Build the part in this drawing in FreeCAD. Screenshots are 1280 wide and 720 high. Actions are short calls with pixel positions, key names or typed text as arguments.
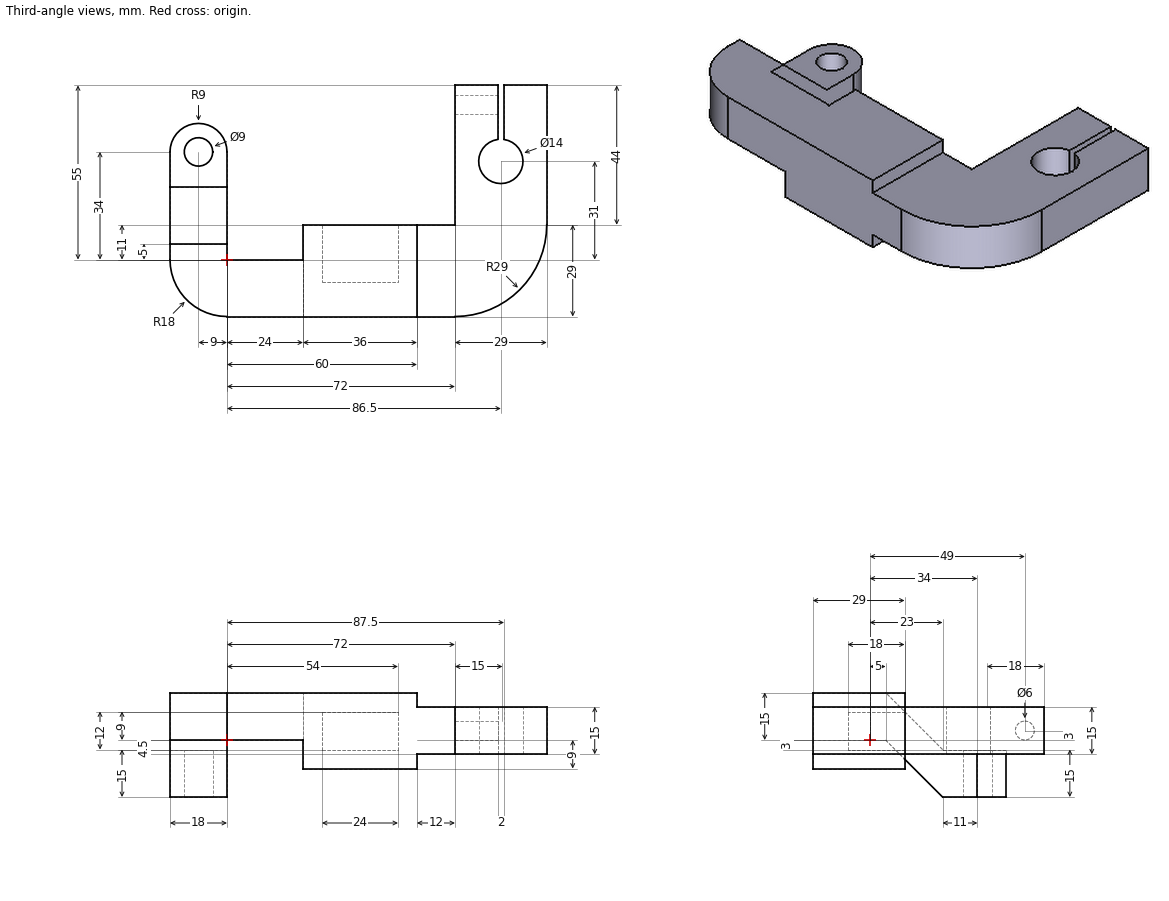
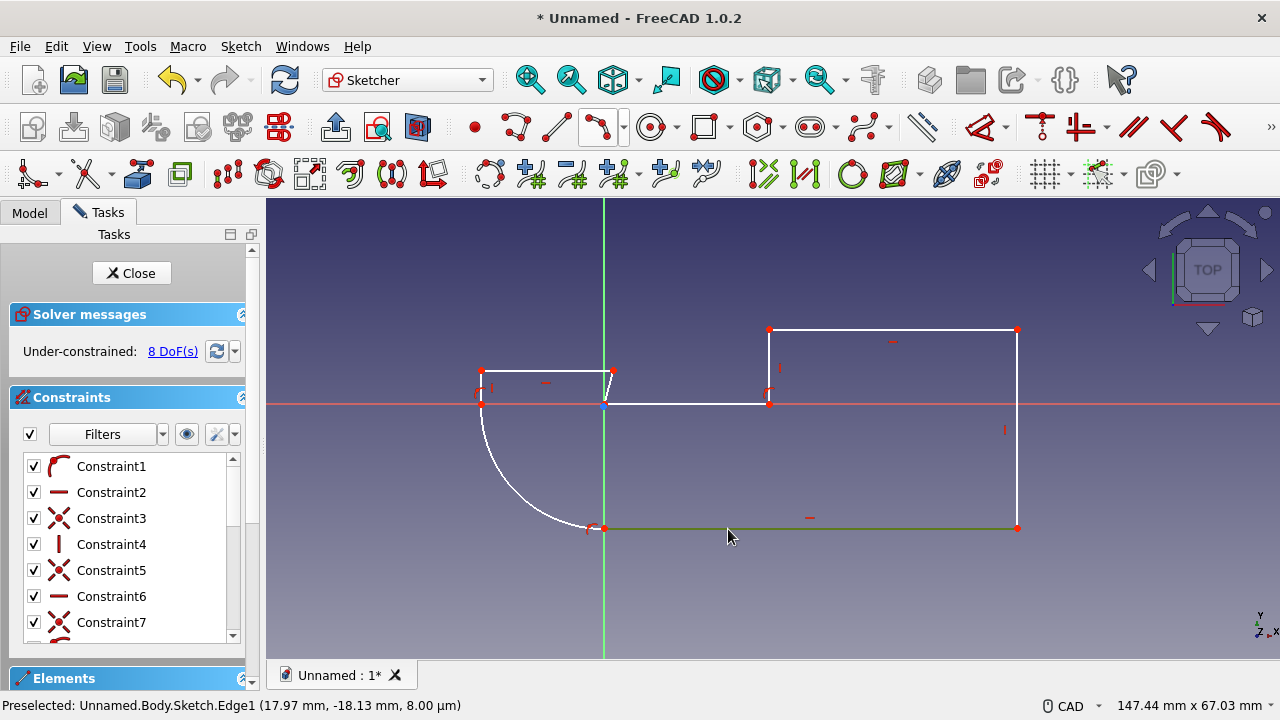
click(494, 461)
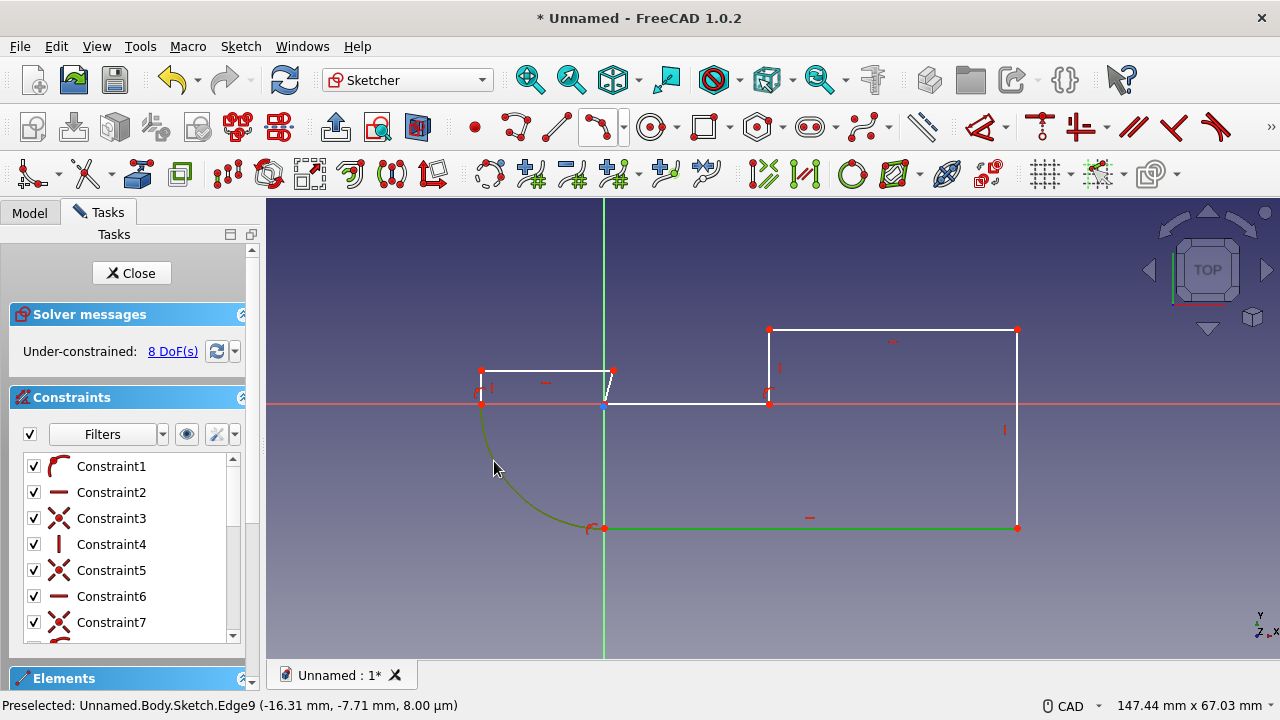
click(1216, 128)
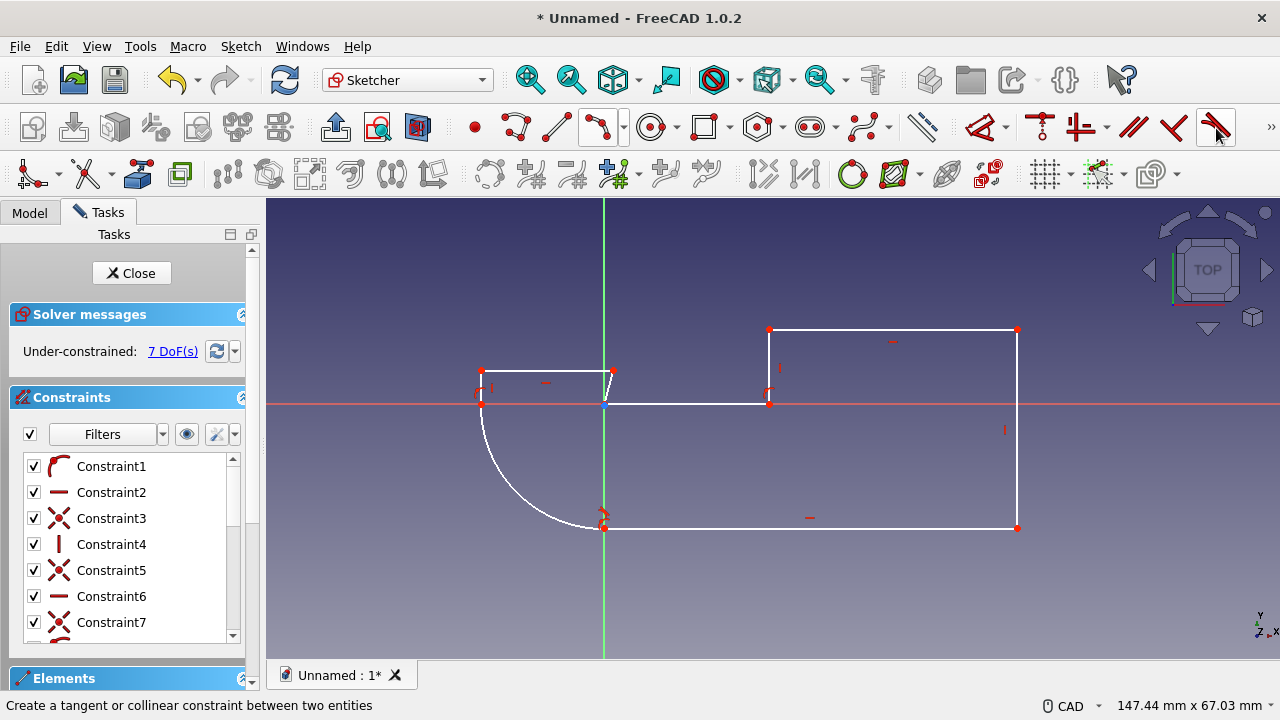
scroll(481, 381, up, 2)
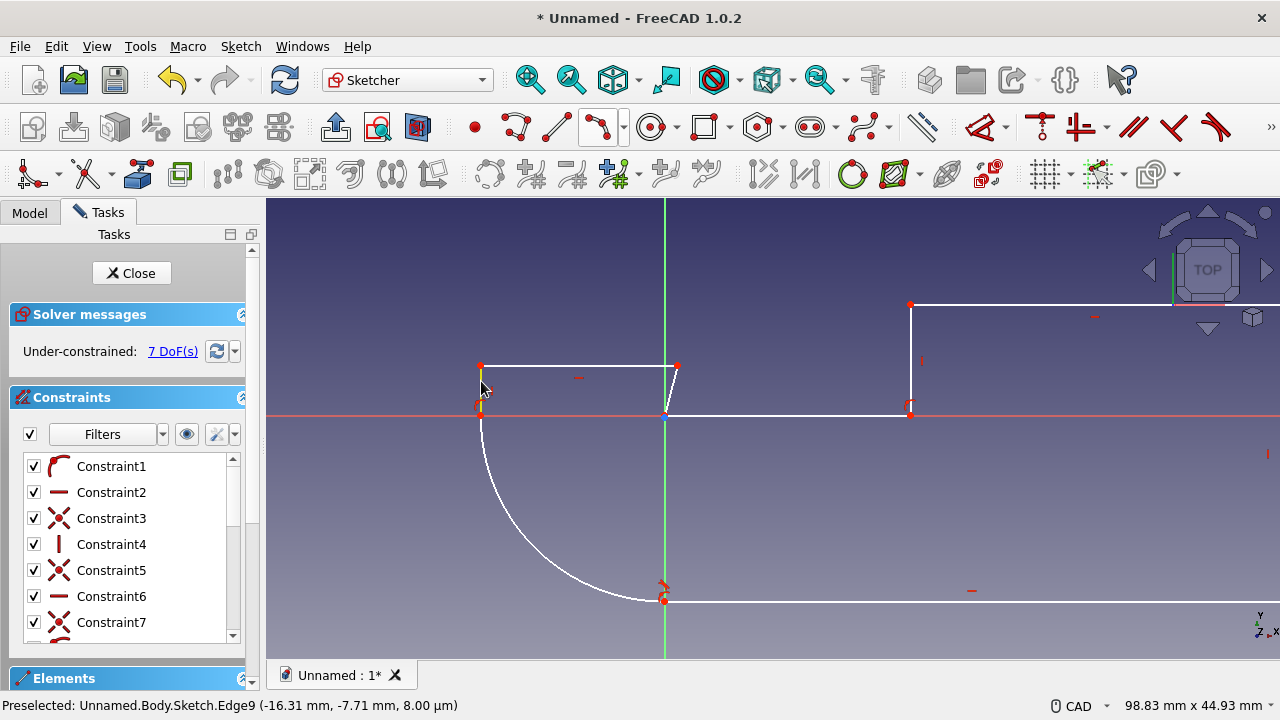
click(481, 381)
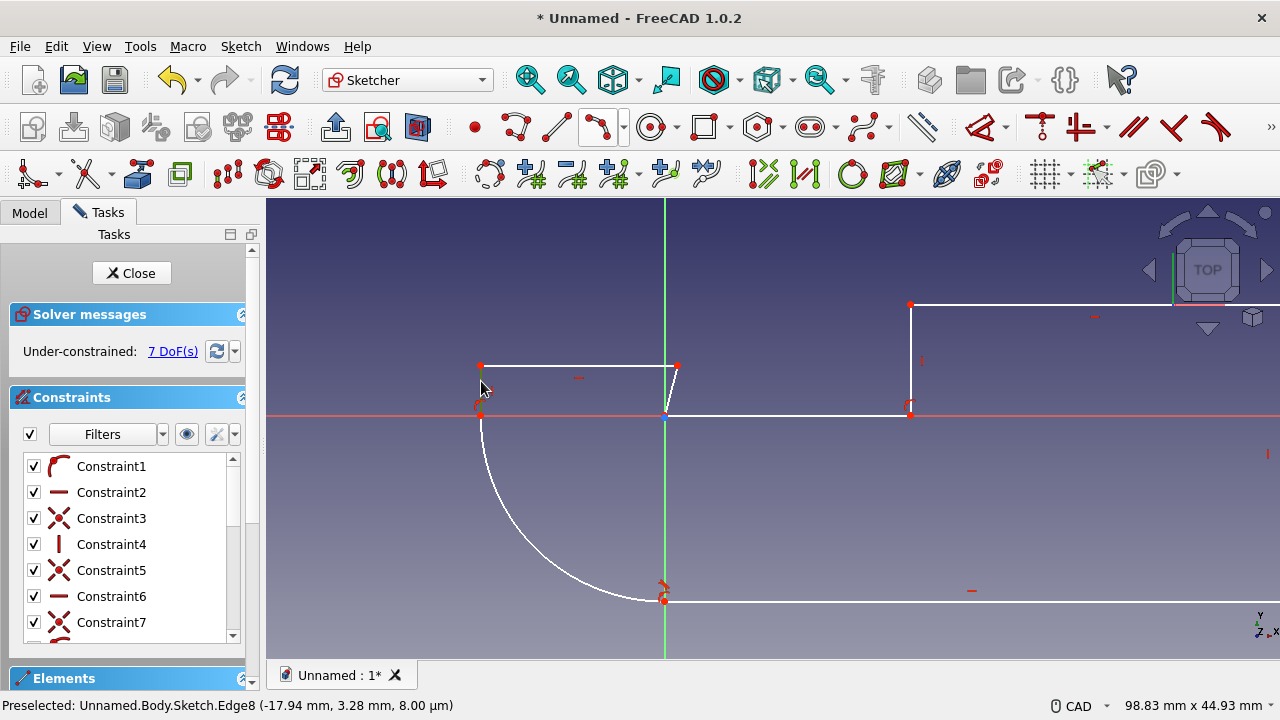
click(500, 500)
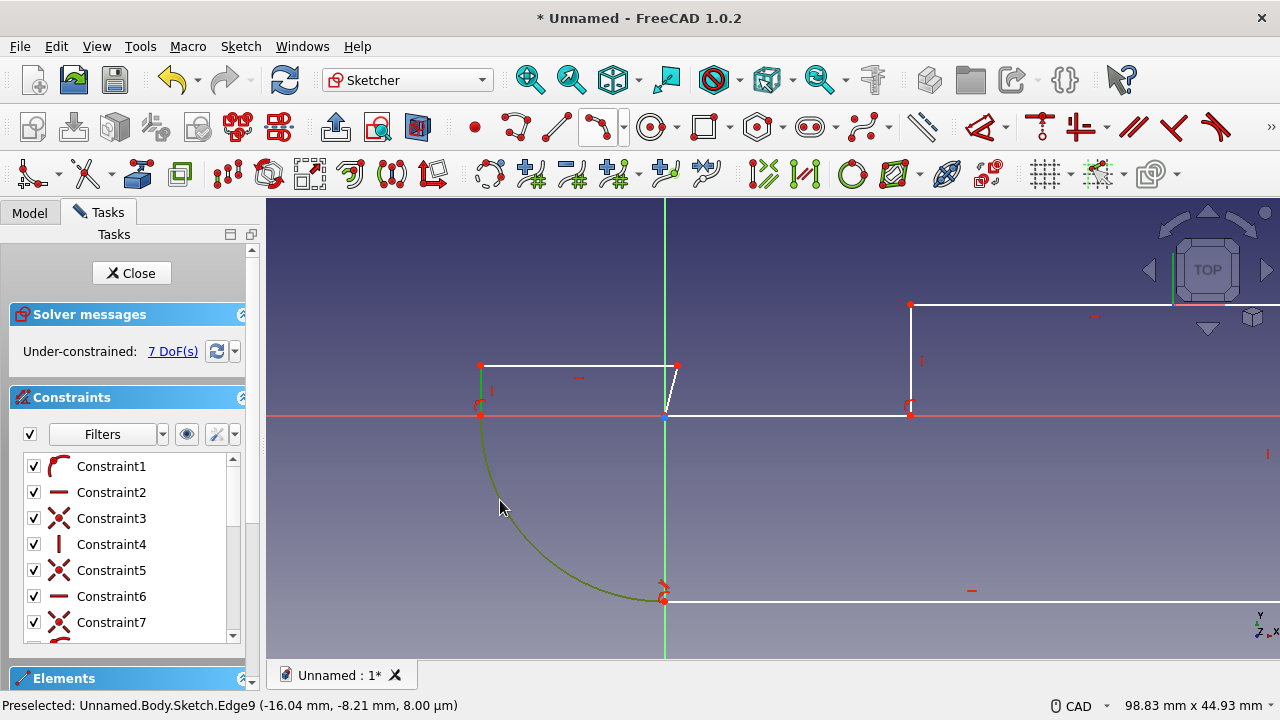
click(1216, 128)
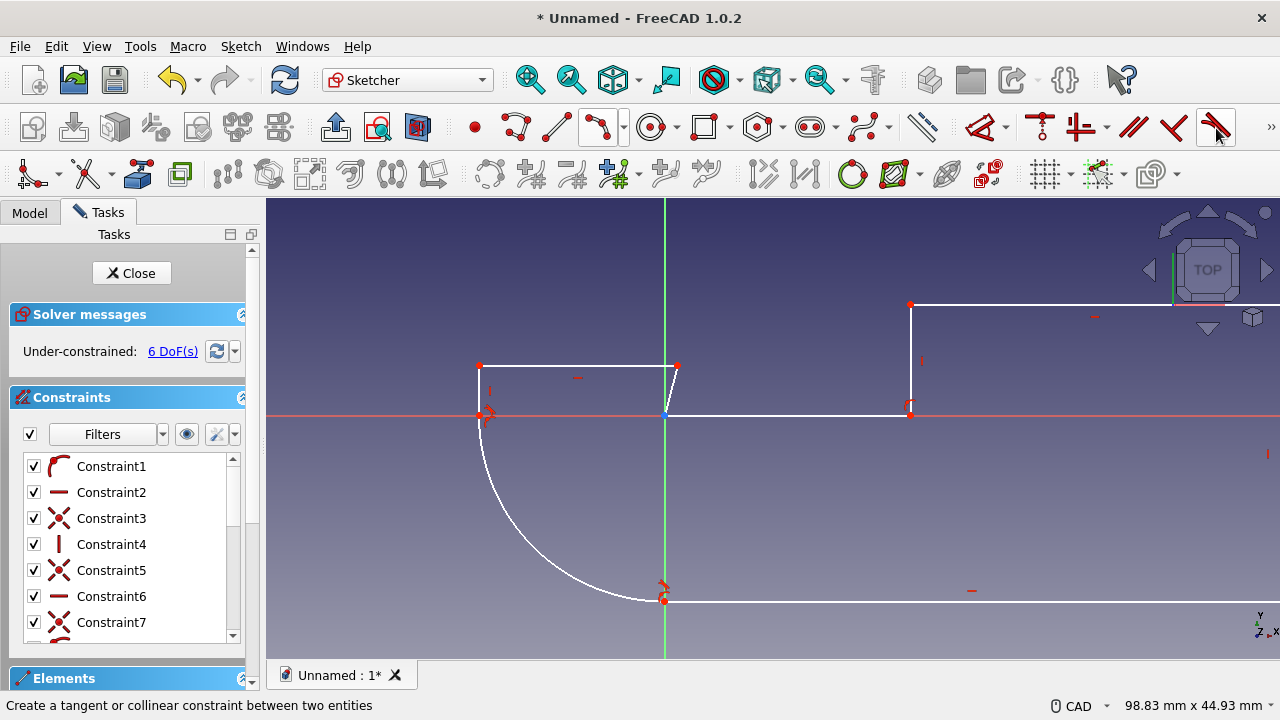
click(669, 401)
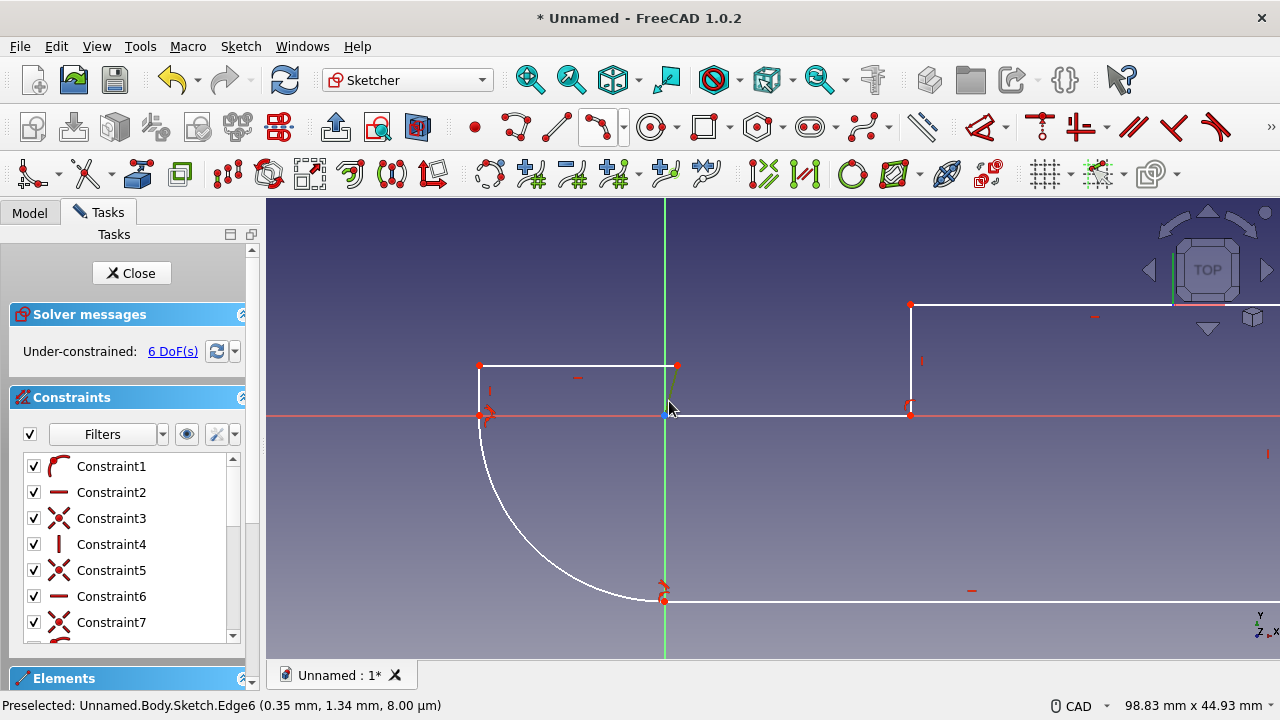
click(1106, 128)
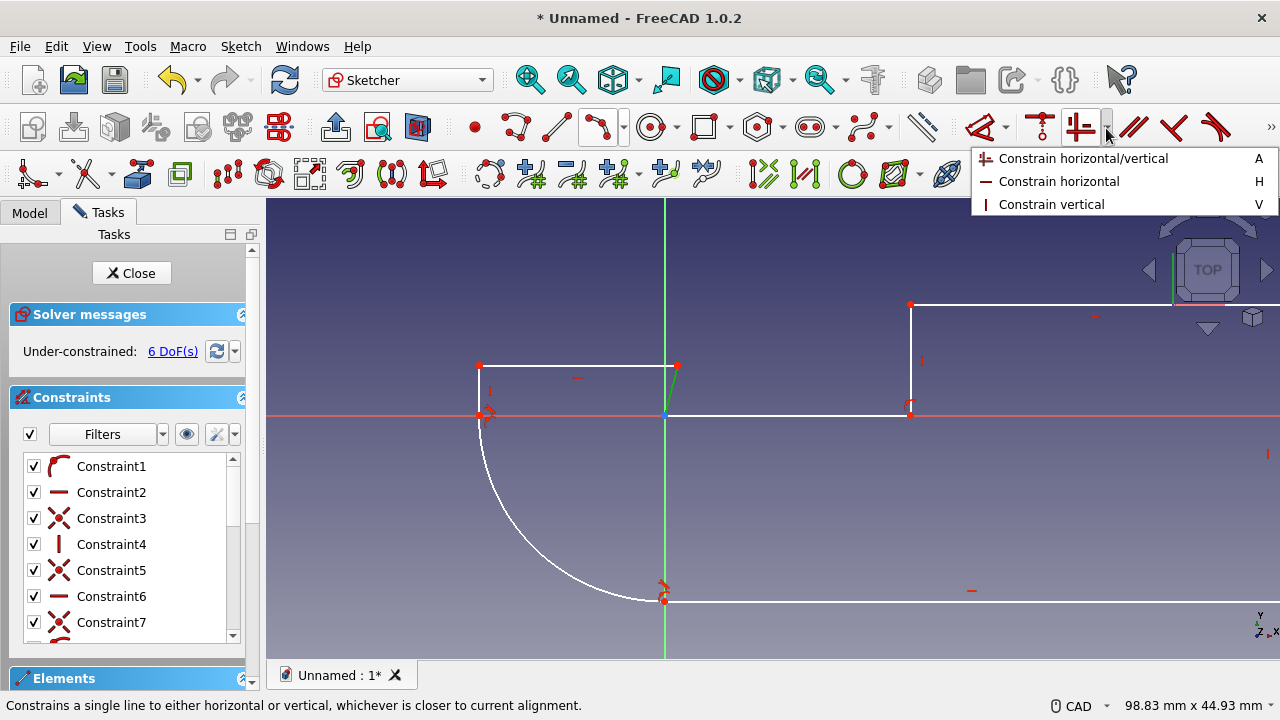
click(1125, 204)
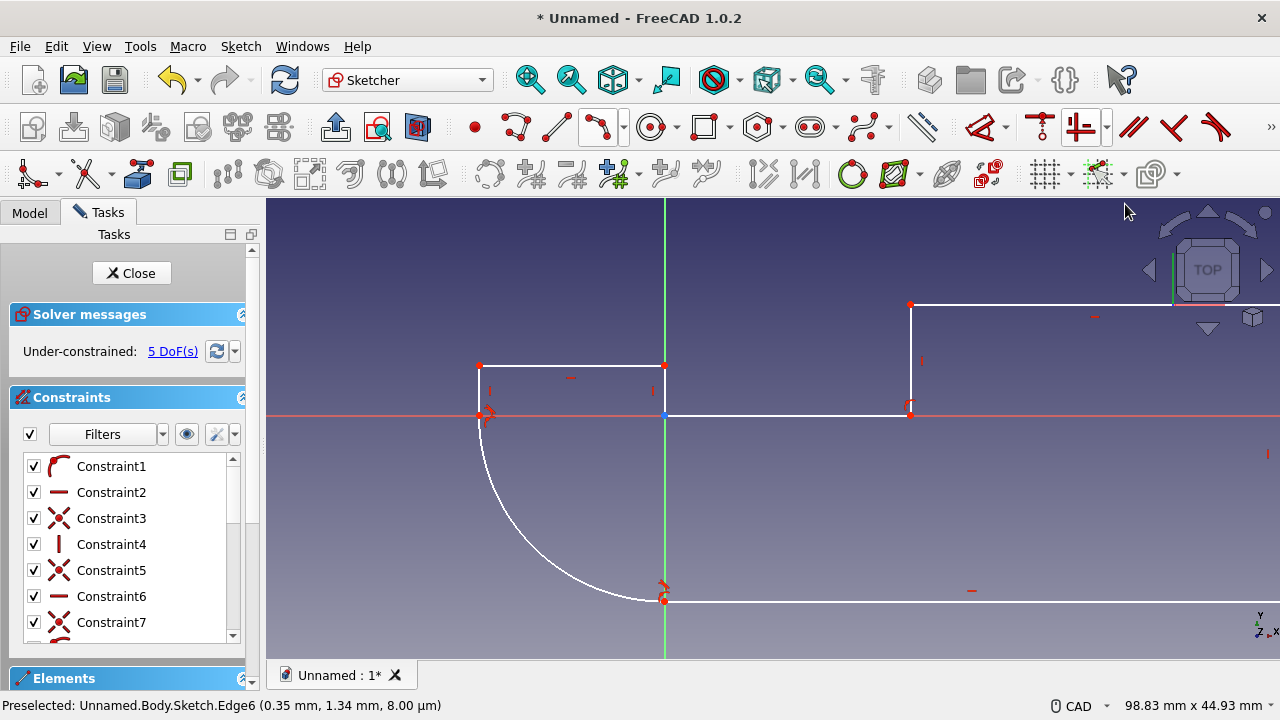
click(980, 128)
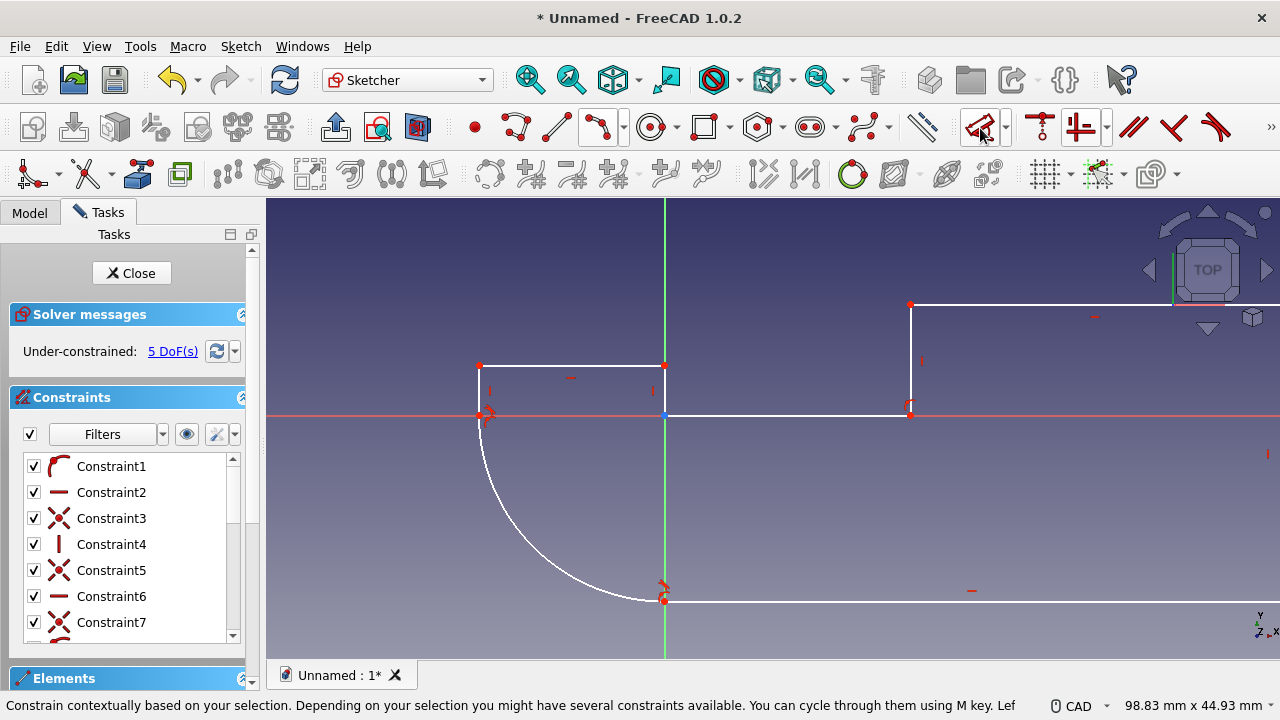
click(499, 500)
click(470, 515)